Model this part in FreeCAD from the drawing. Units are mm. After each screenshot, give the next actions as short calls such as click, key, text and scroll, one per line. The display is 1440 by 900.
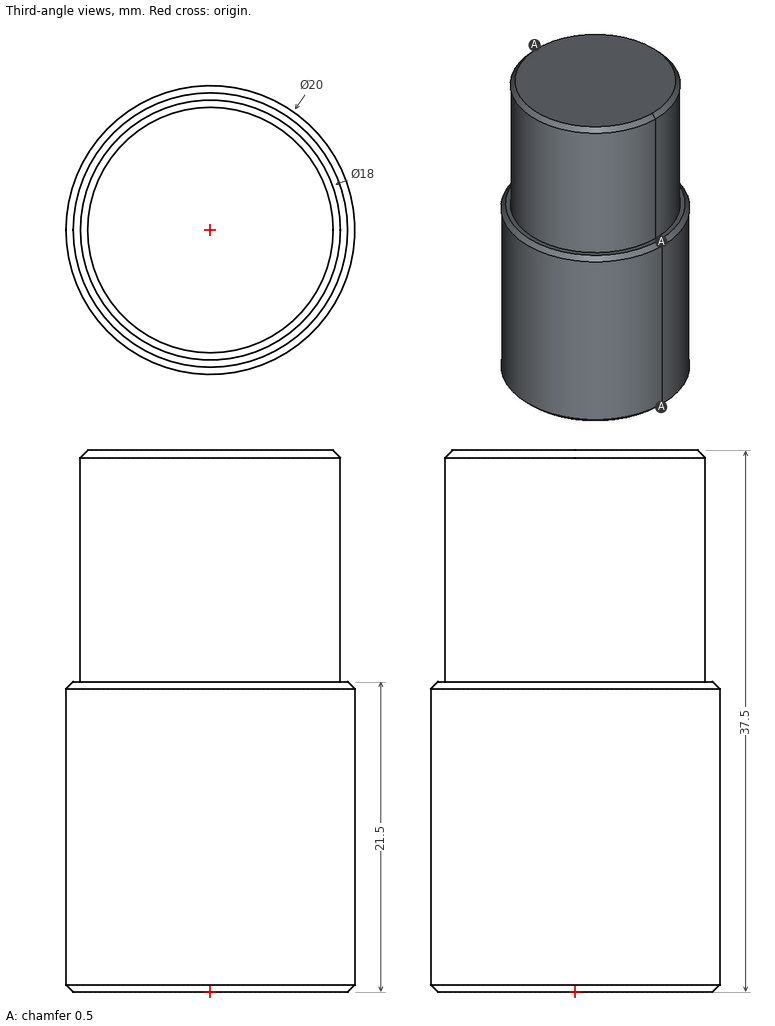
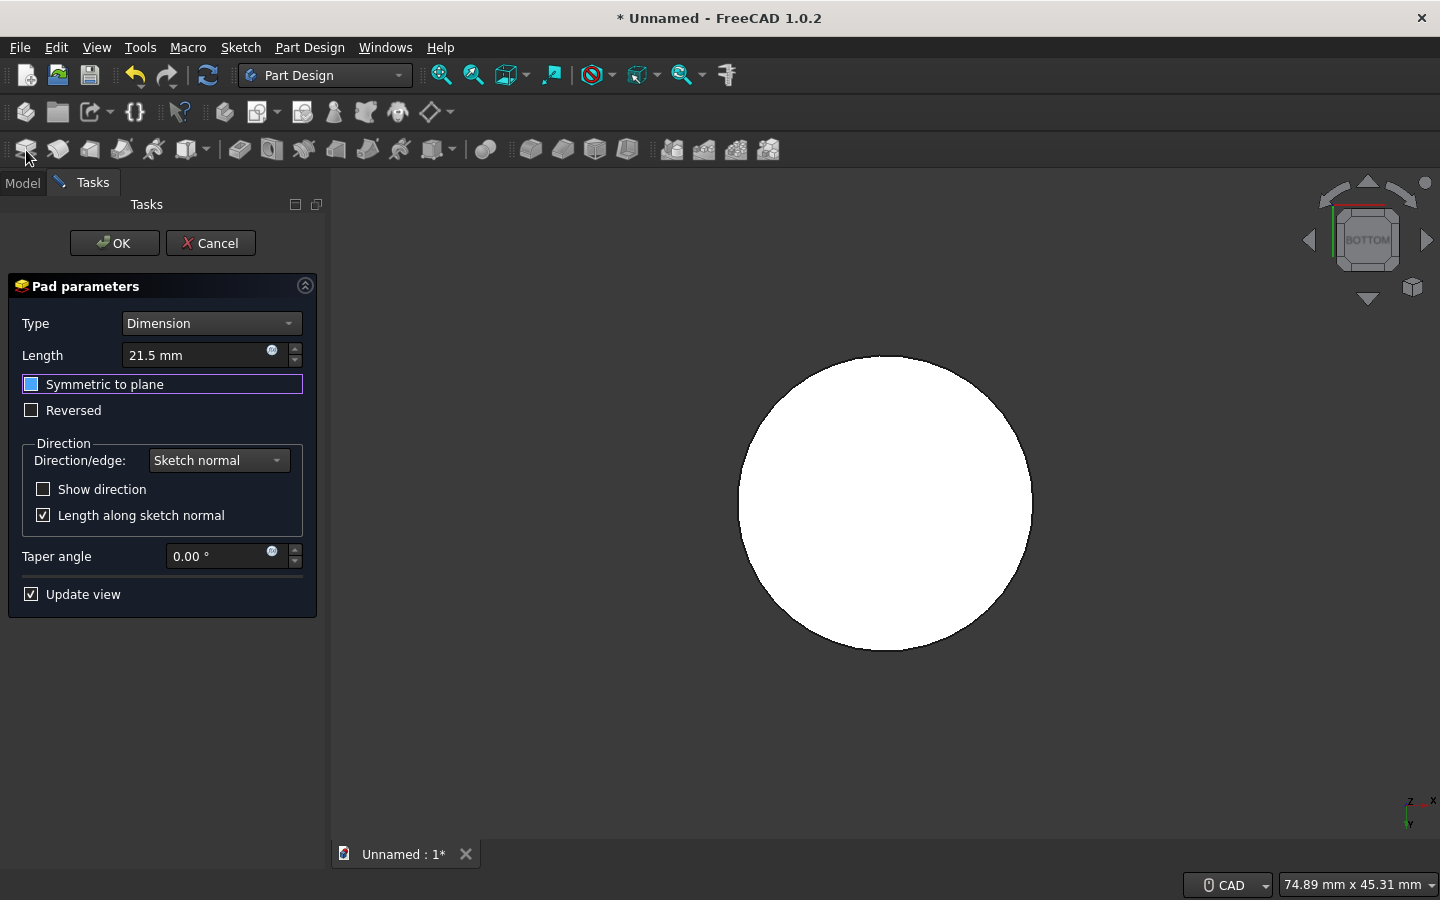
click(30, 410)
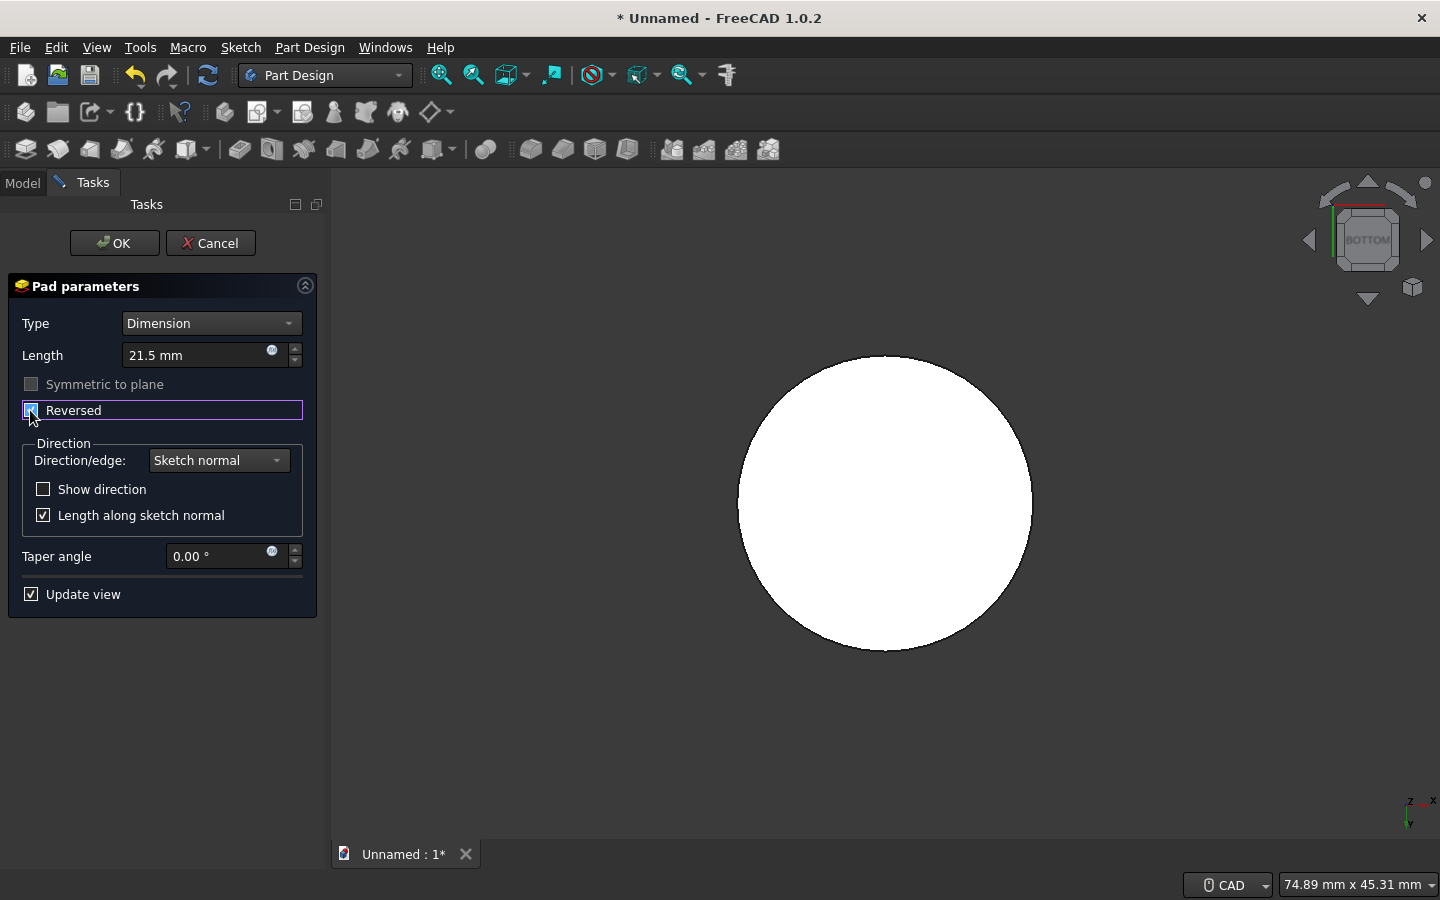
click(115, 243)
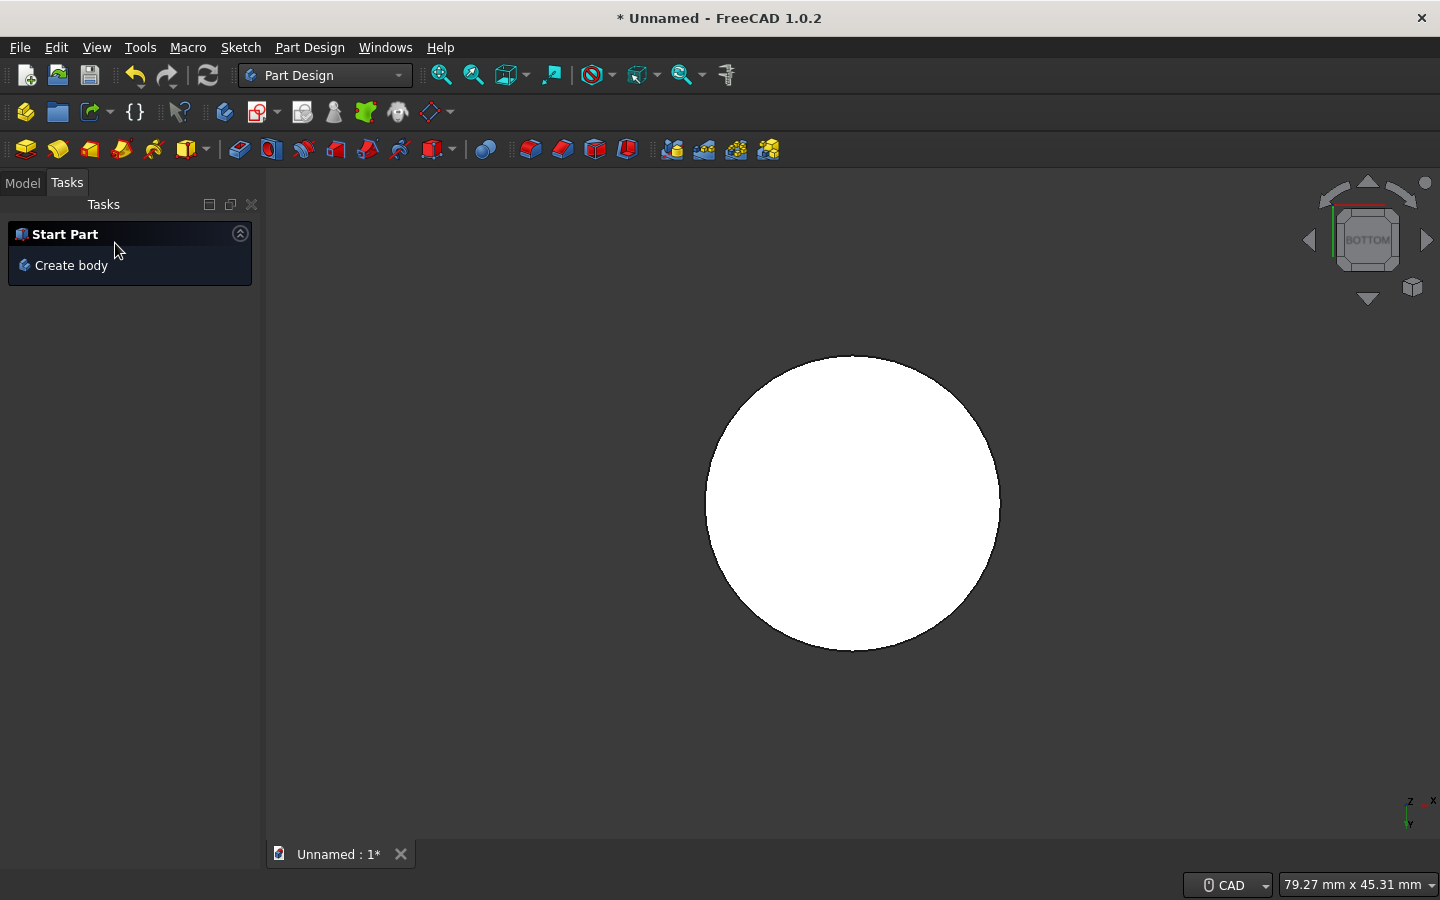
click(442, 76)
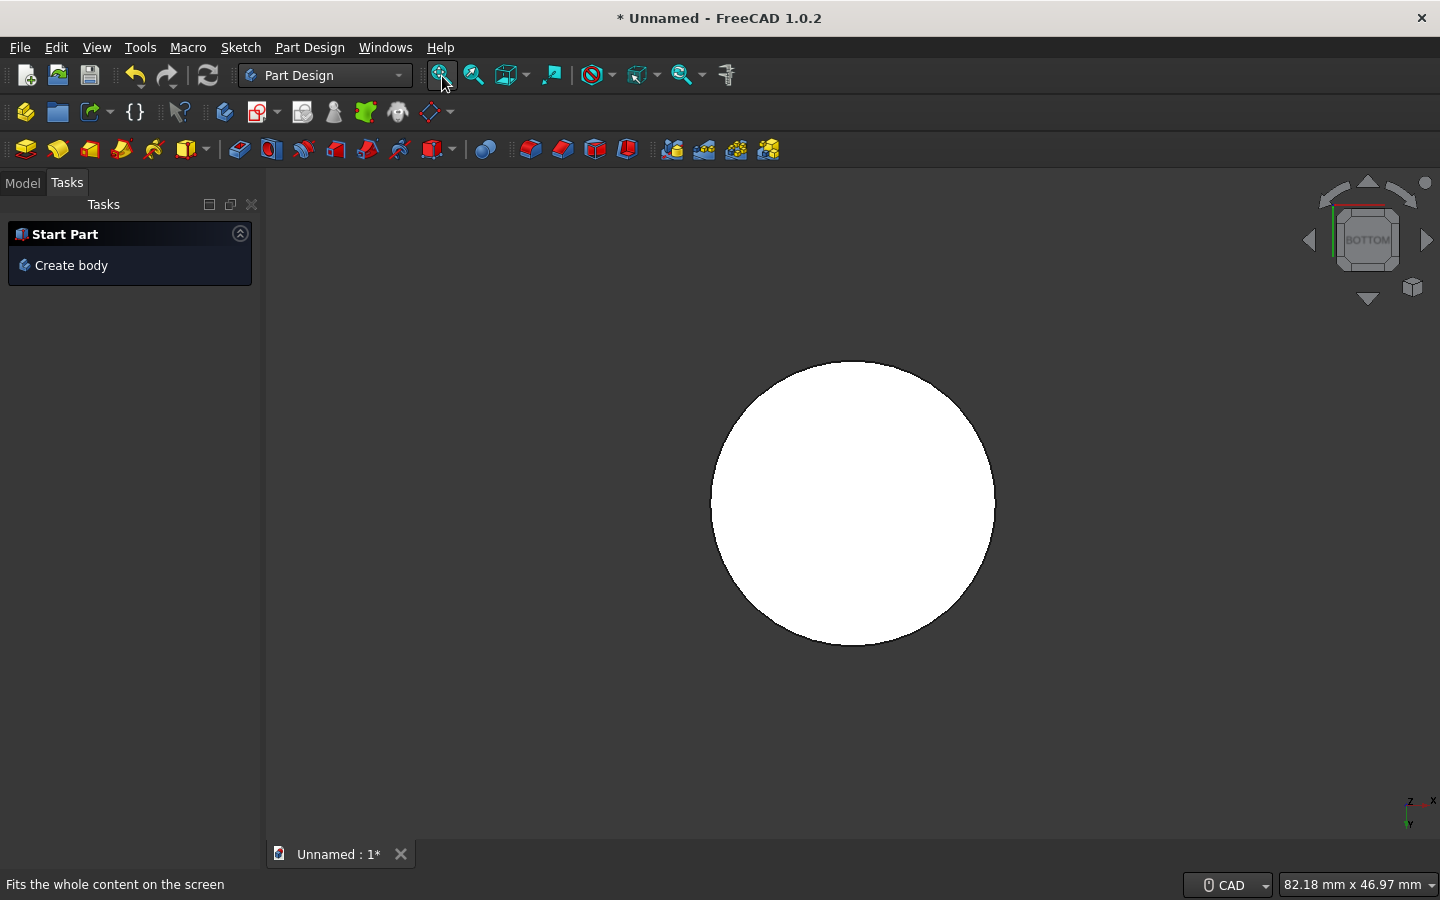
click(710, 502)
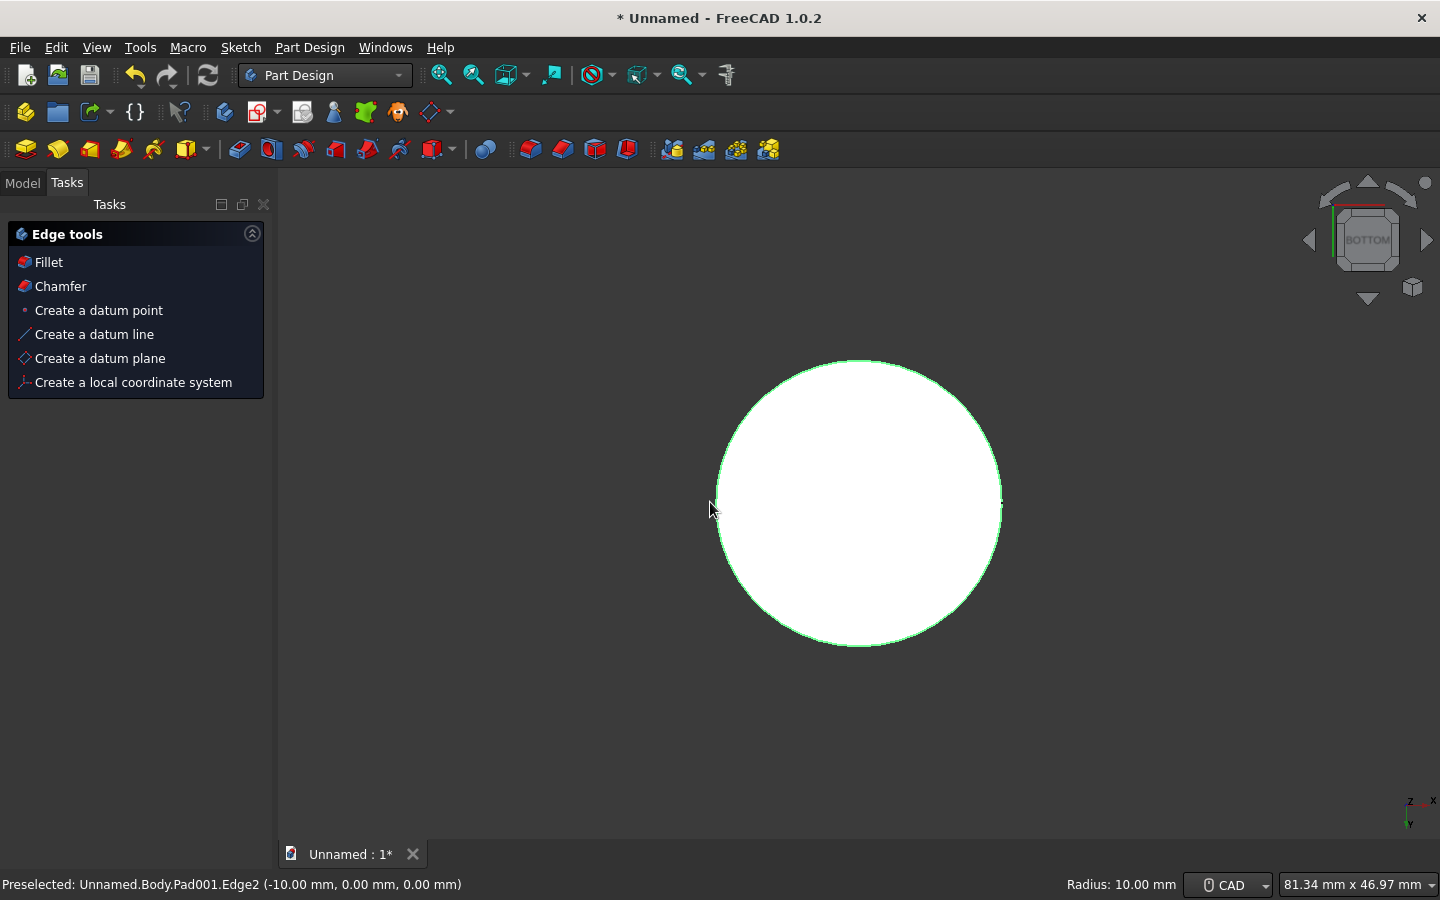
key(0)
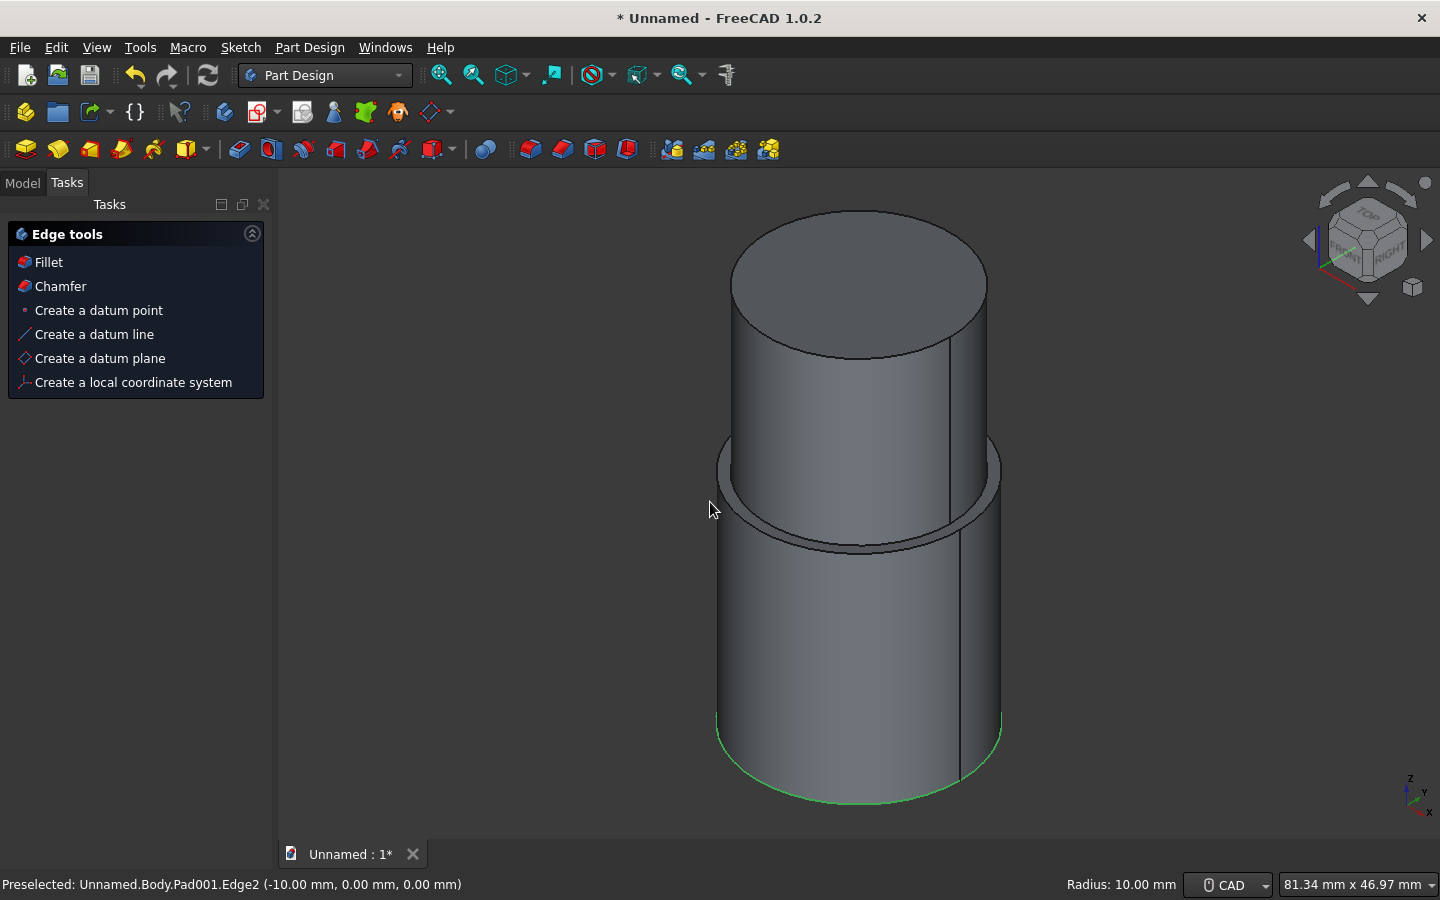
click(442, 76)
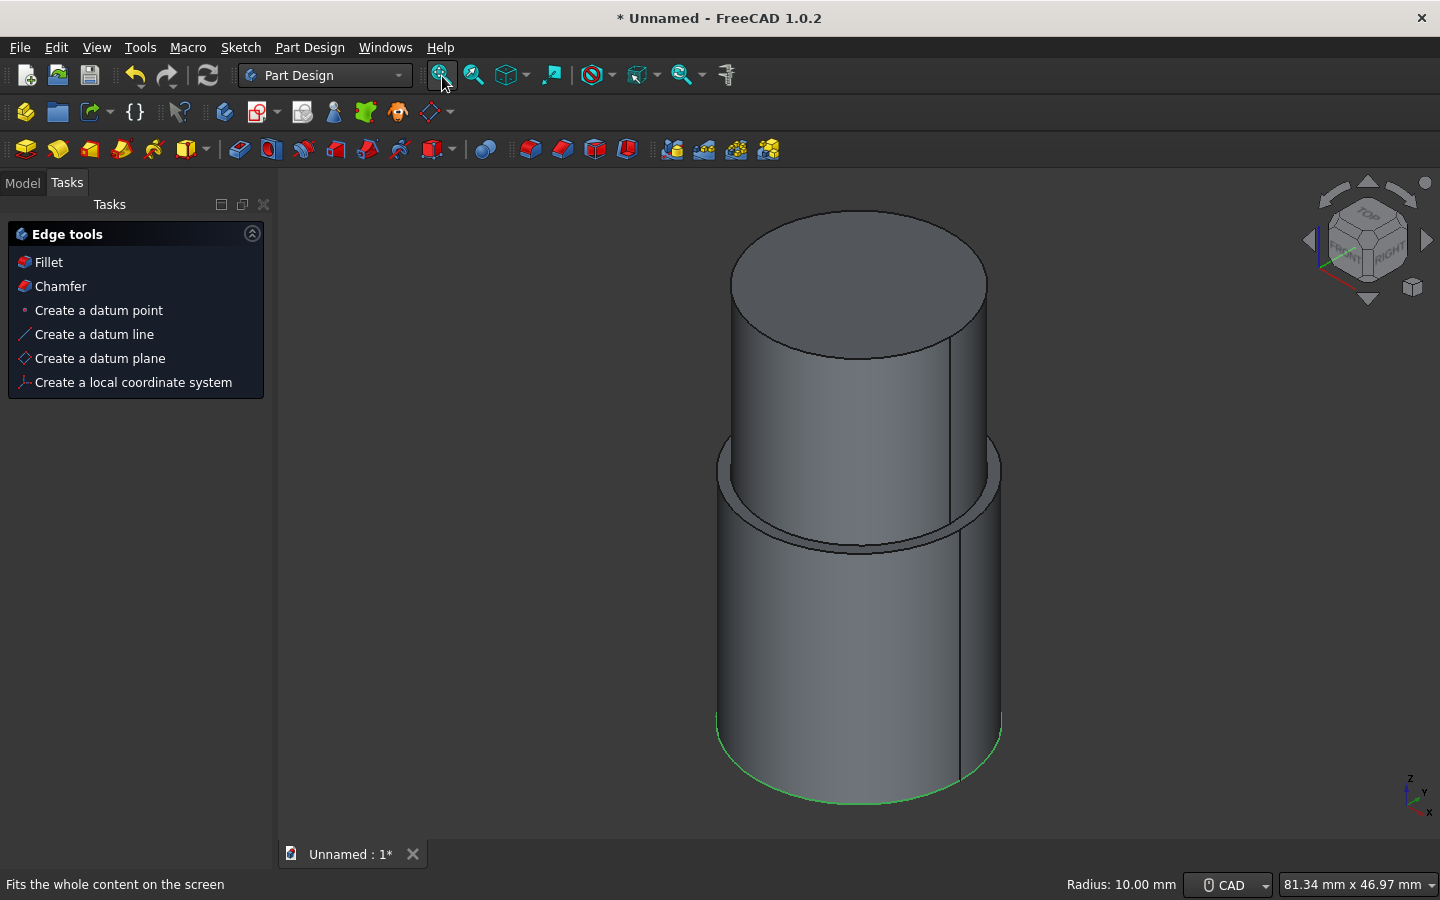
click(744, 317, ctrl)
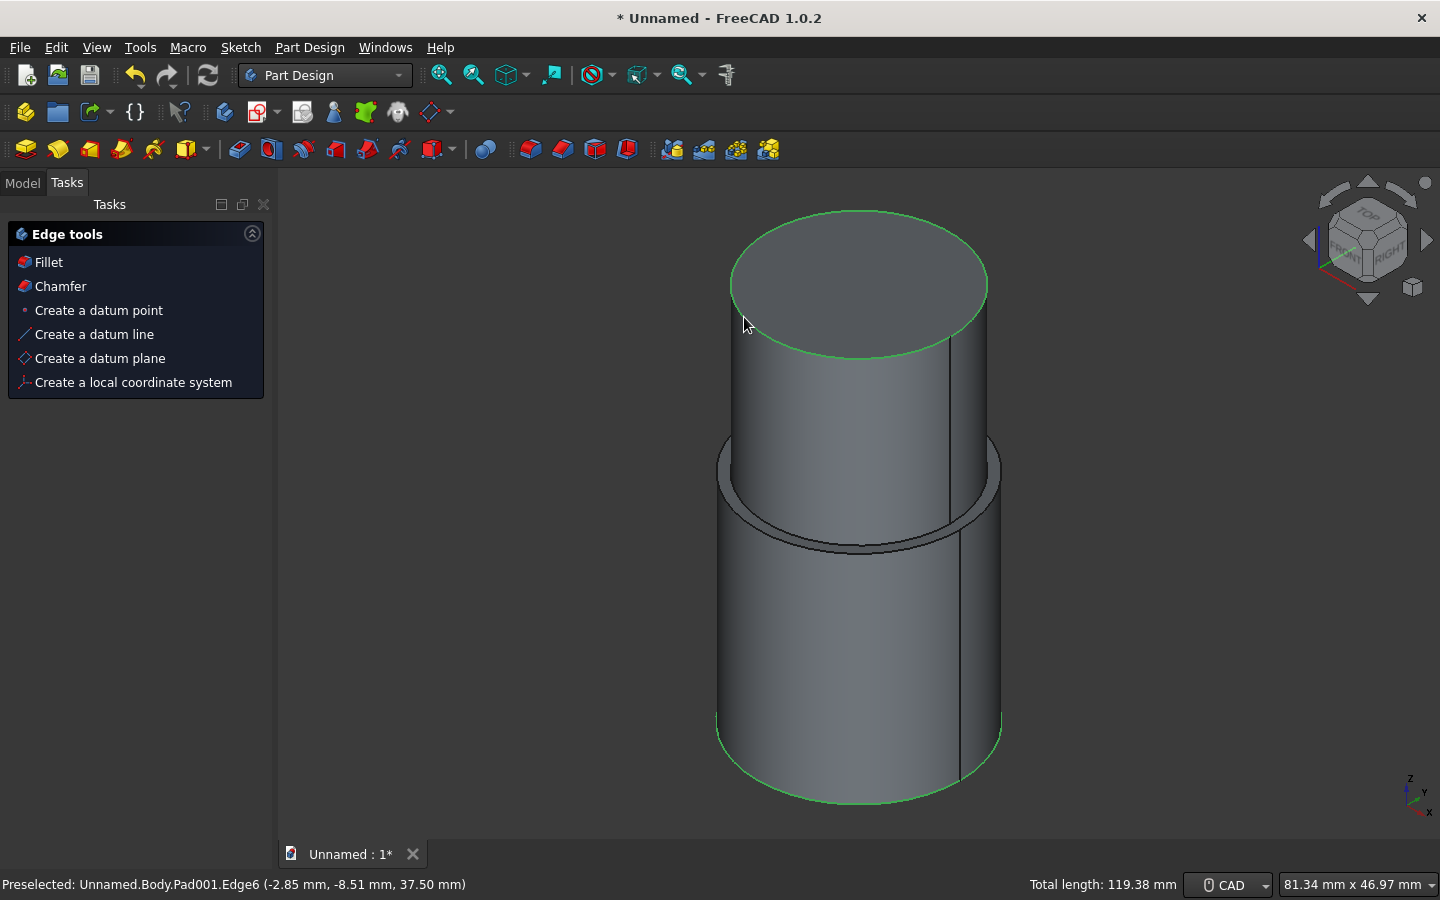
click(732, 508, ctrl)